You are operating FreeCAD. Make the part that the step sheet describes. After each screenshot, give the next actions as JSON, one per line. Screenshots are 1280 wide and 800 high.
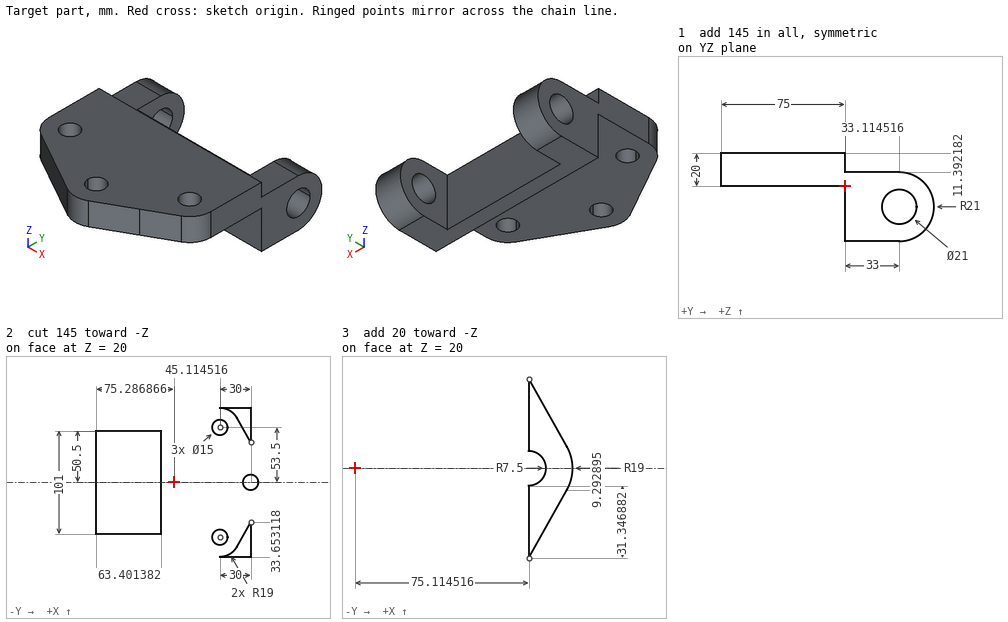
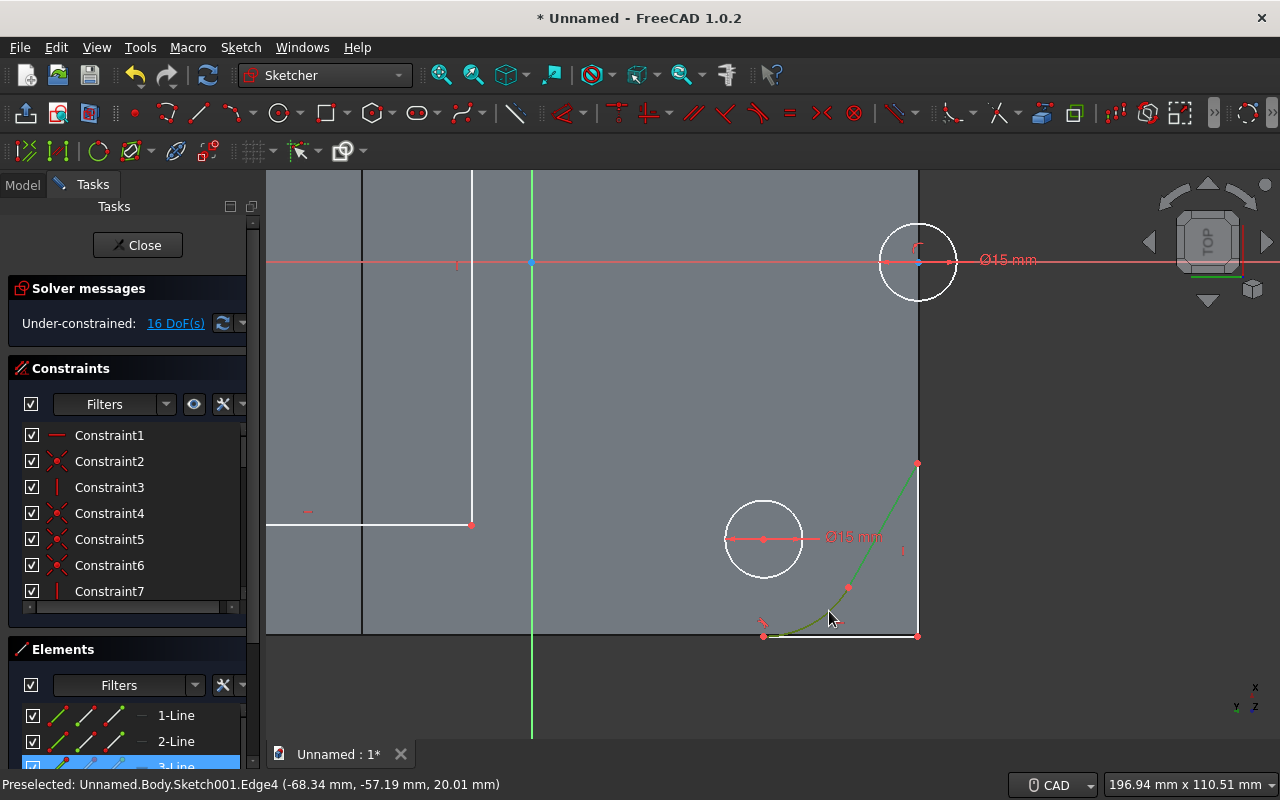
{"action": "left_click", "coordinate": [758, 114]}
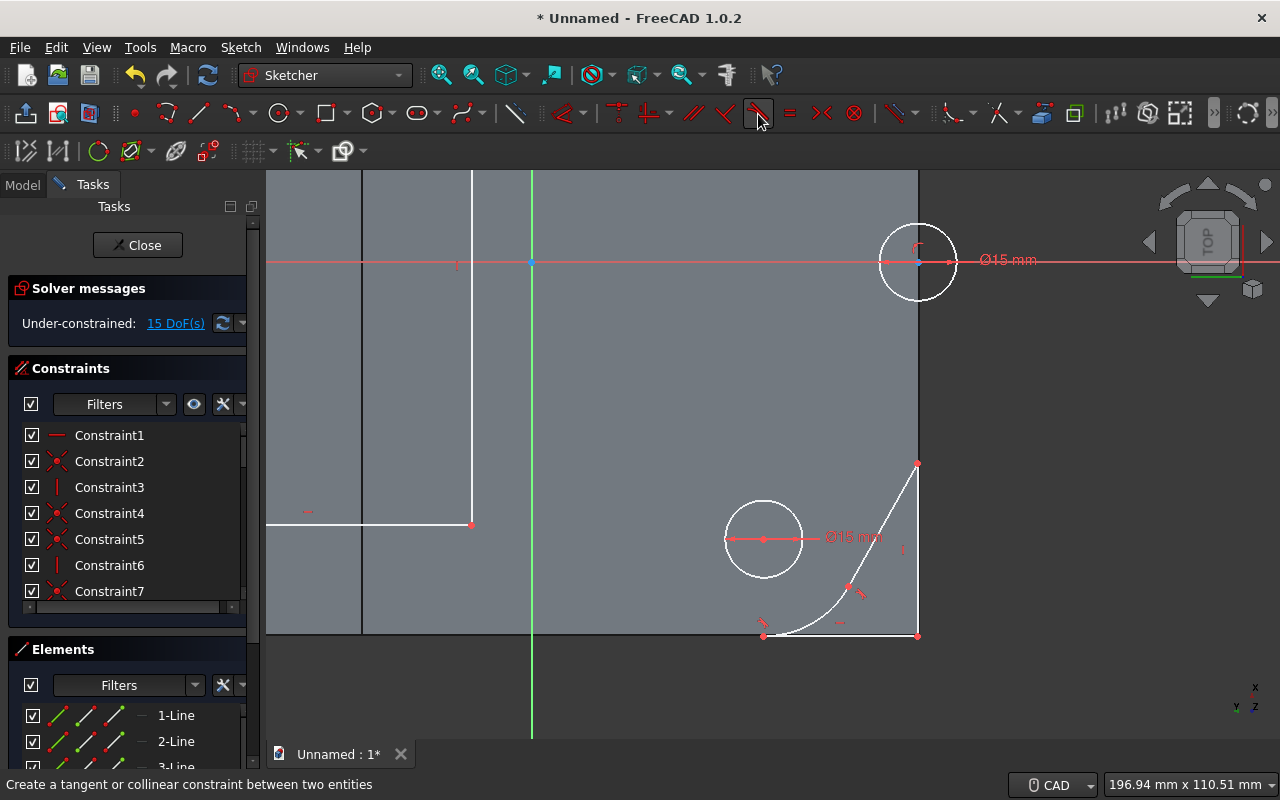
{"action": "scroll", "coordinate": [830, 611], "scroll_direction": "down", "scroll_amount": 4}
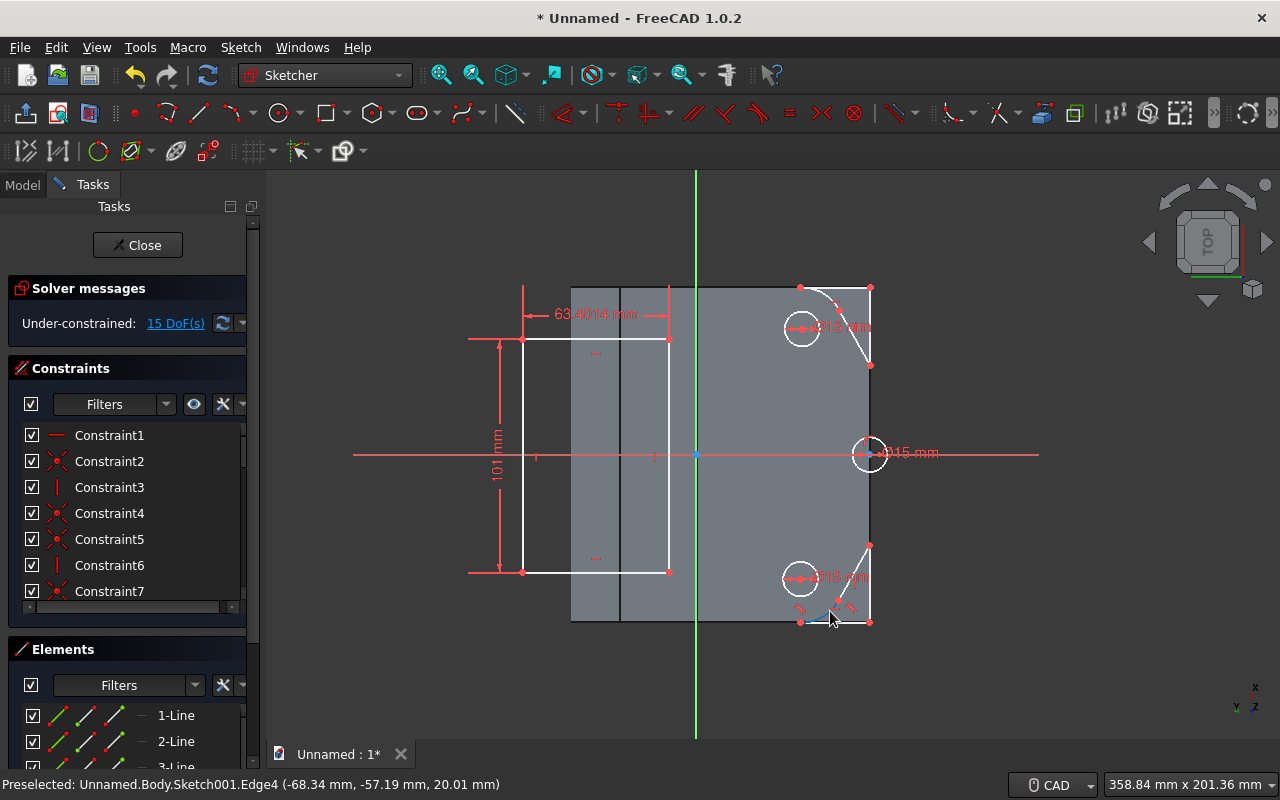
{"action": "left_click", "coordinate": [861, 349]}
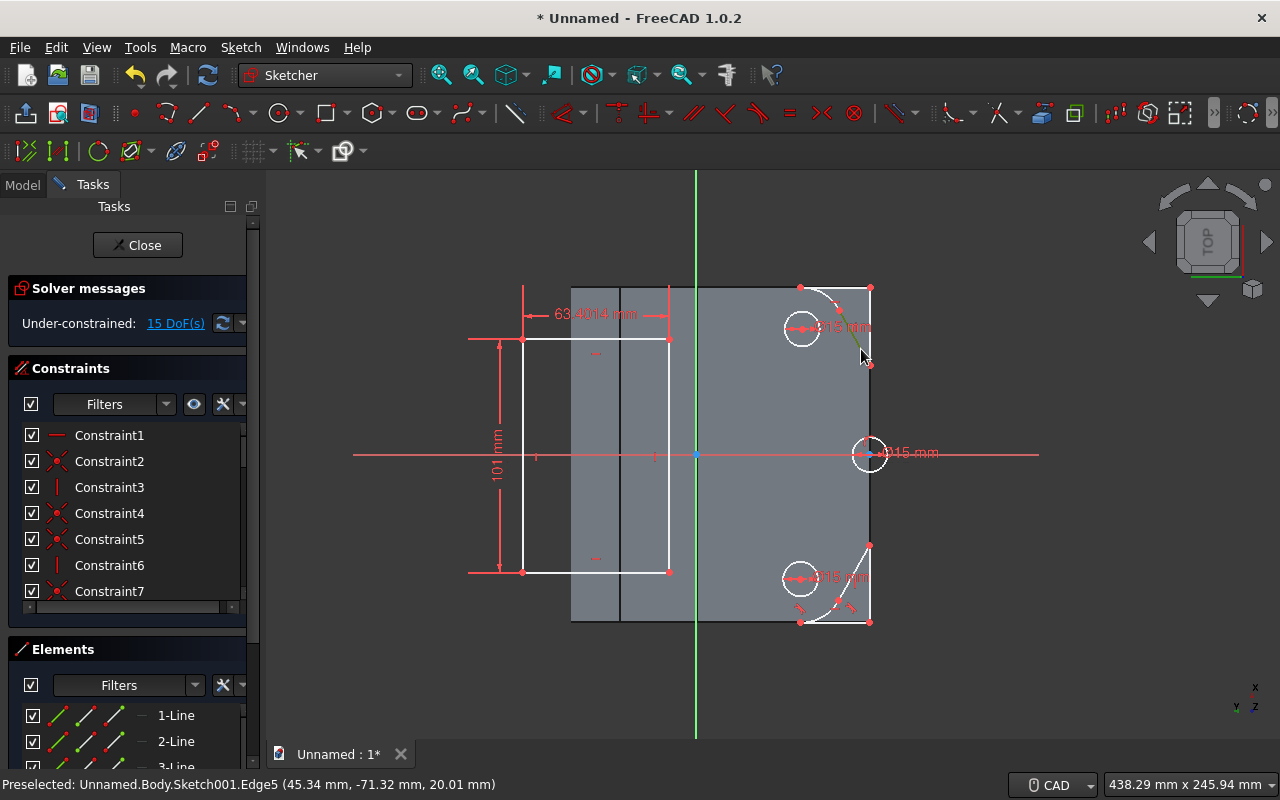
{"action": "left_click", "coordinate": [823, 293]}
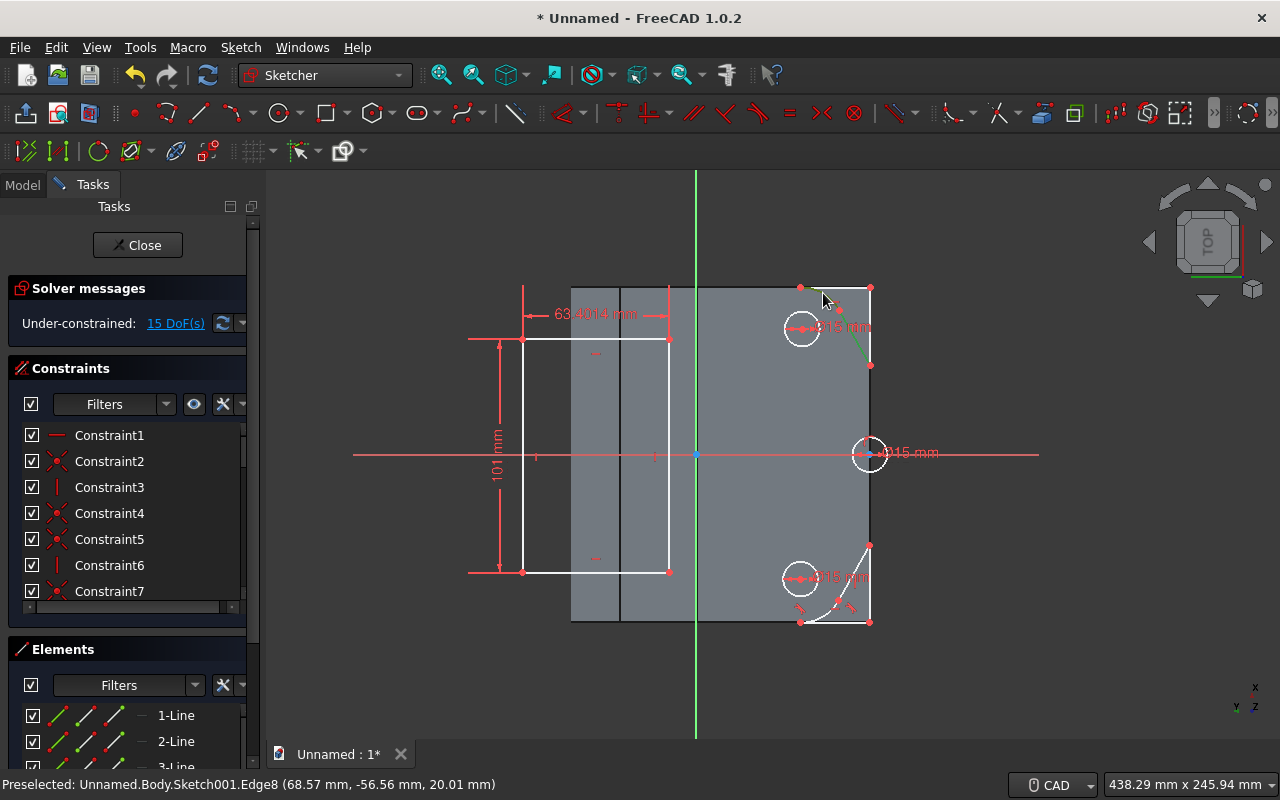
{"action": "left_click", "coordinate": [758, 114]}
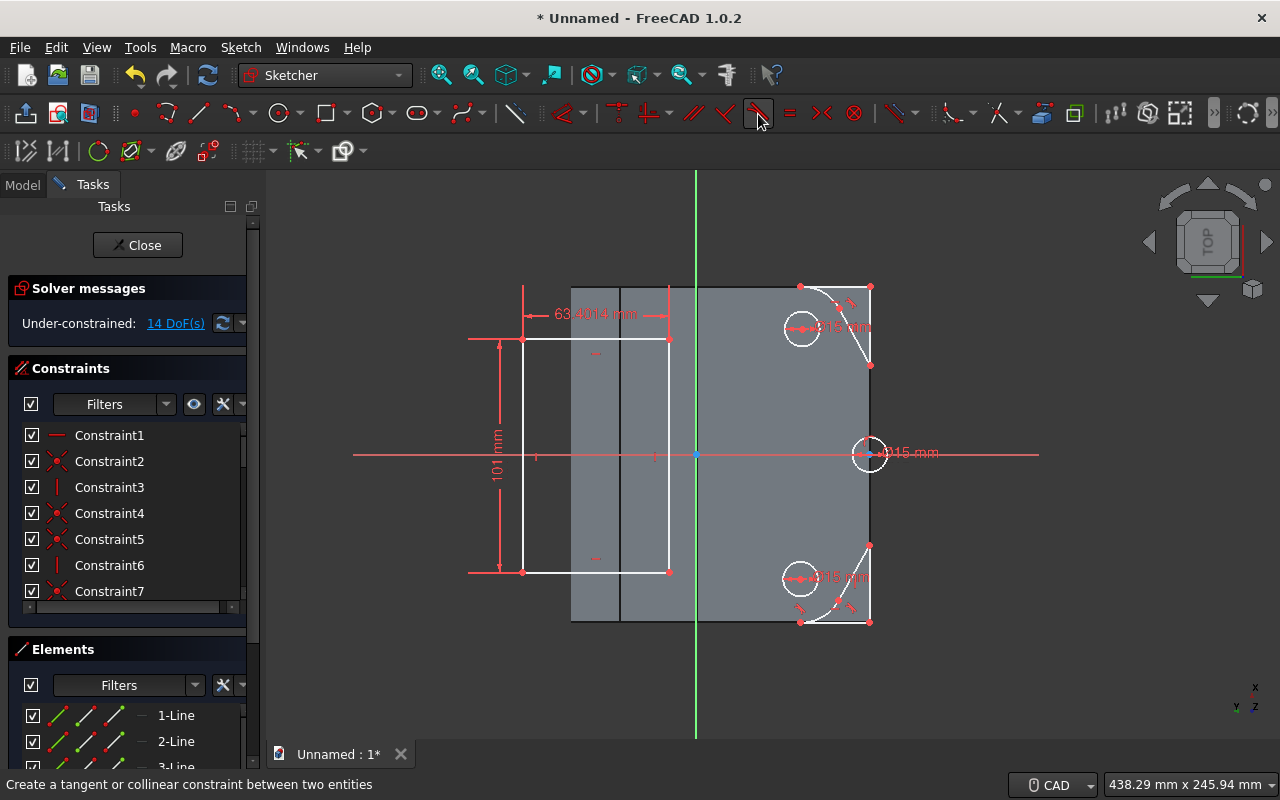
{"action": "left_click", "coordinate": [849, 287]}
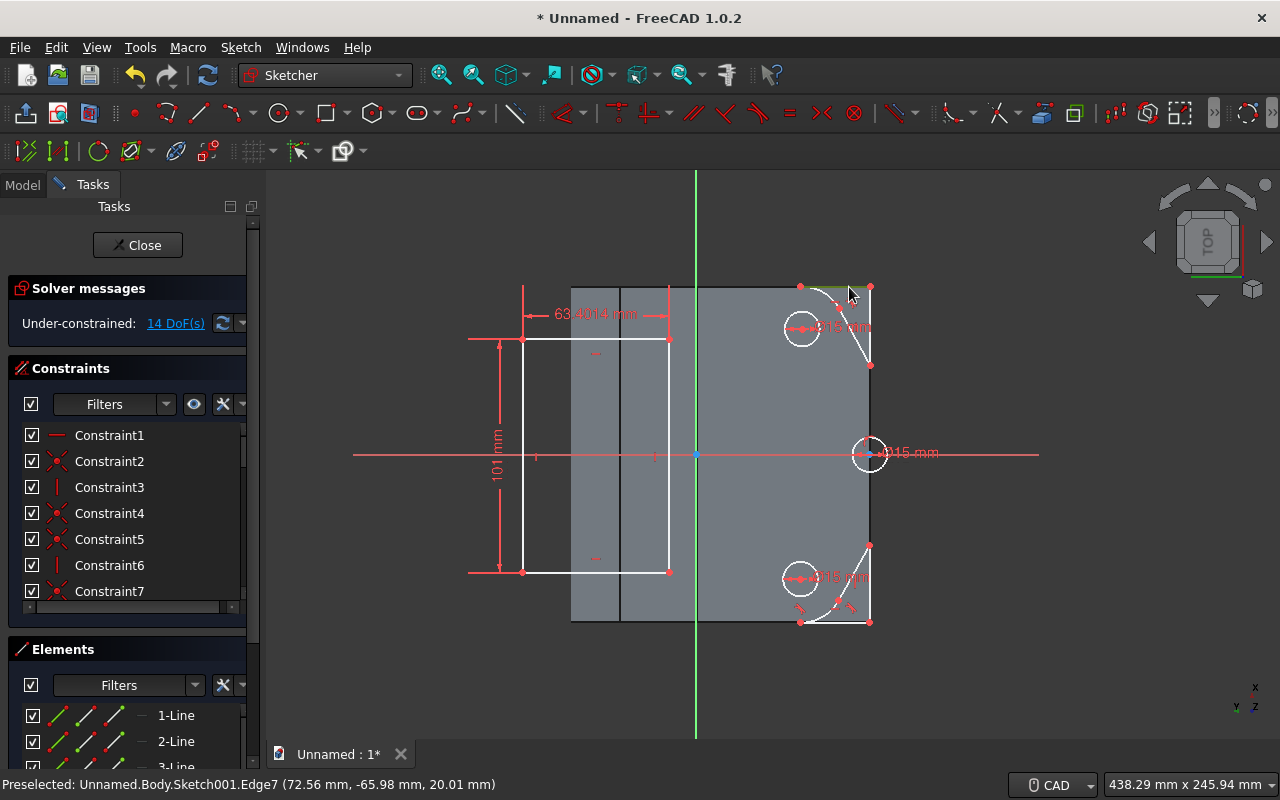
{"action": "scroll", "coordinate": [831, 298], "scroll_direction": "up", "scroll_amount": 2}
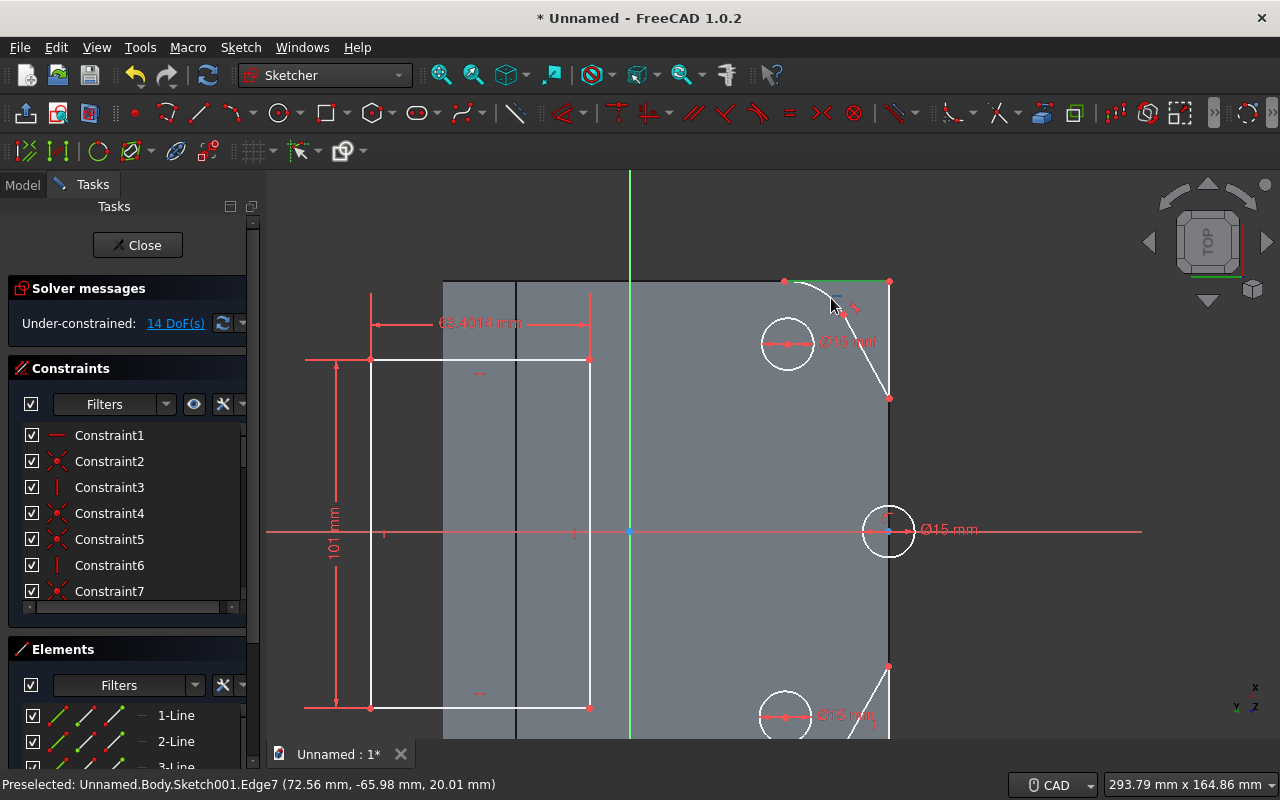
{"action": "left_click", "coordinate": [830, 297]}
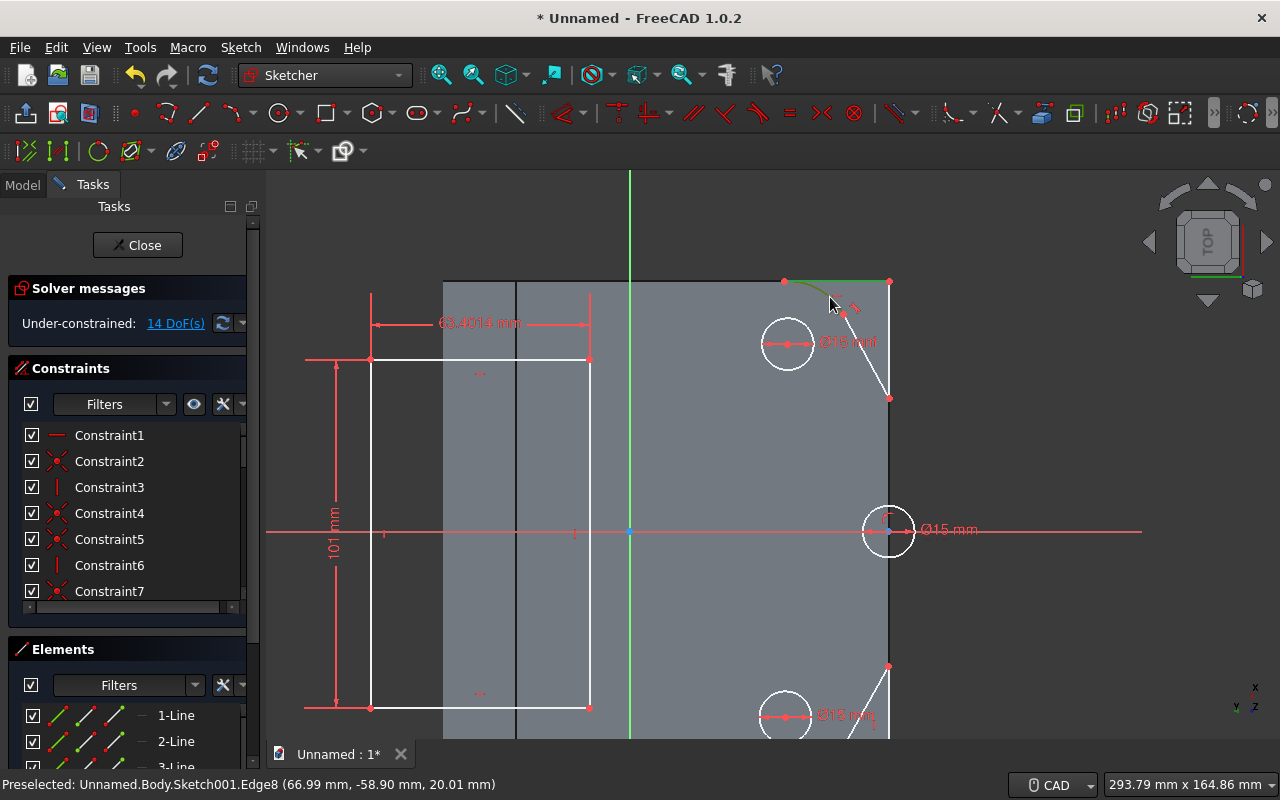
{"action": "left_click", "coordinate": [758, 114]}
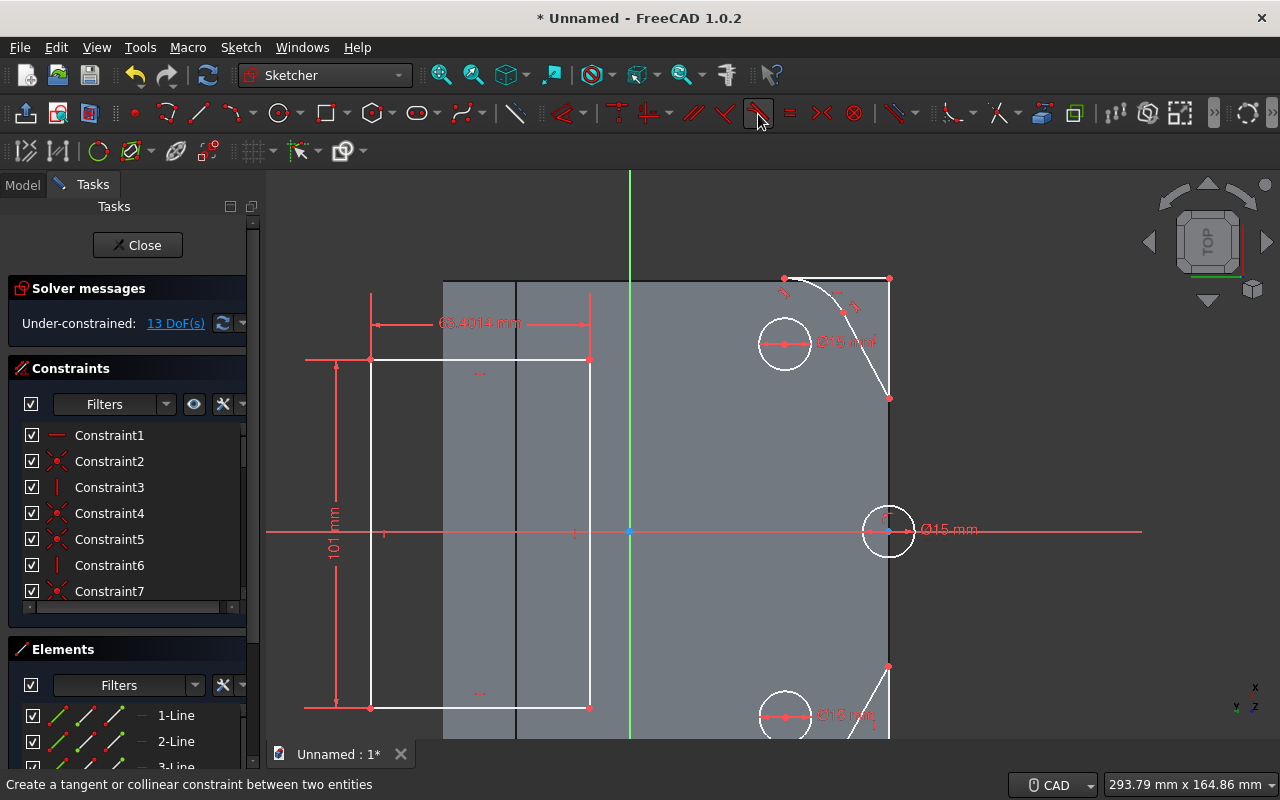
{"action": "scroll", "coordinate": [831, 298], "scroll_direction": "down", "scroll_amount": 2}